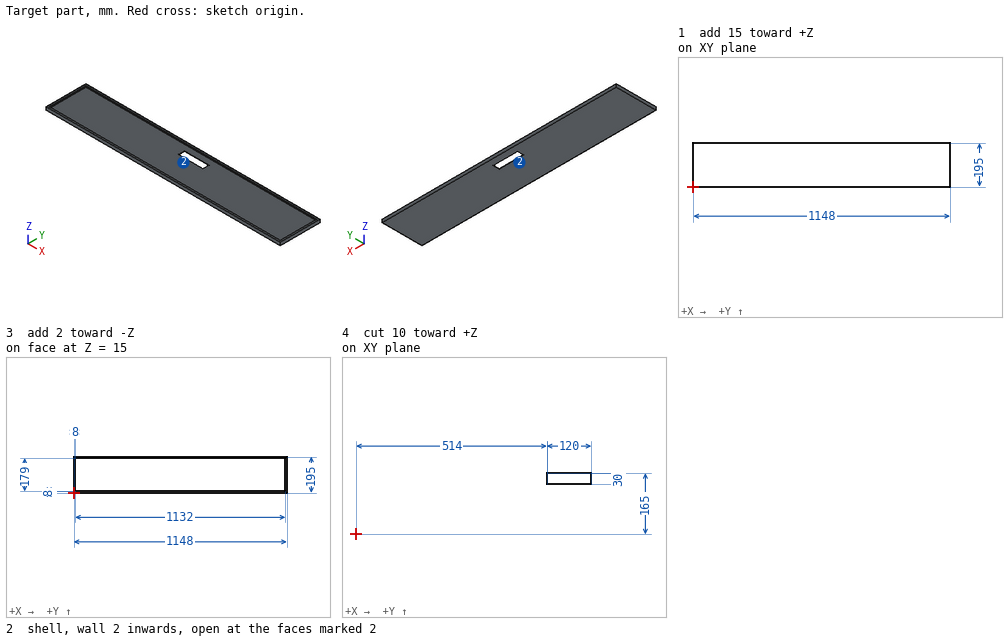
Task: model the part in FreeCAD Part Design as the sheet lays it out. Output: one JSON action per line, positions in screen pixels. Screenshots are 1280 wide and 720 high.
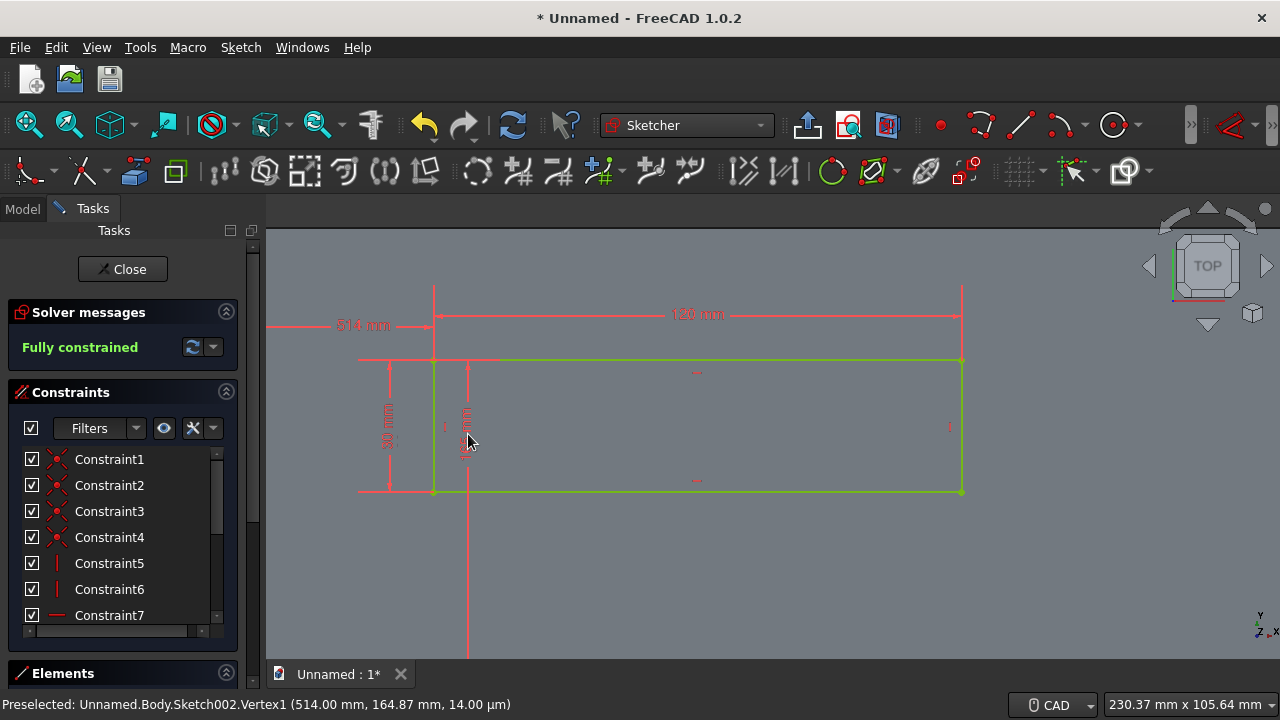
{"action": "left_click", "coordinate": [123, 269]}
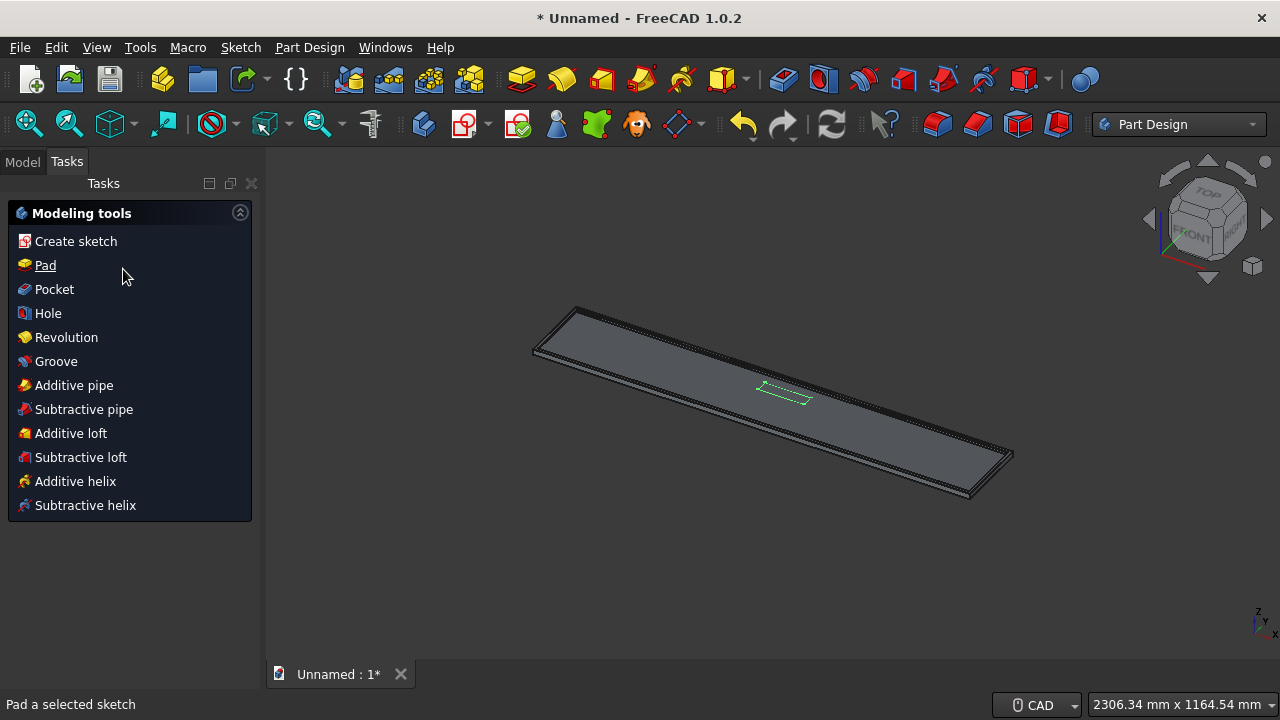
{"action": "left_click", "coordinate": [784, 80]}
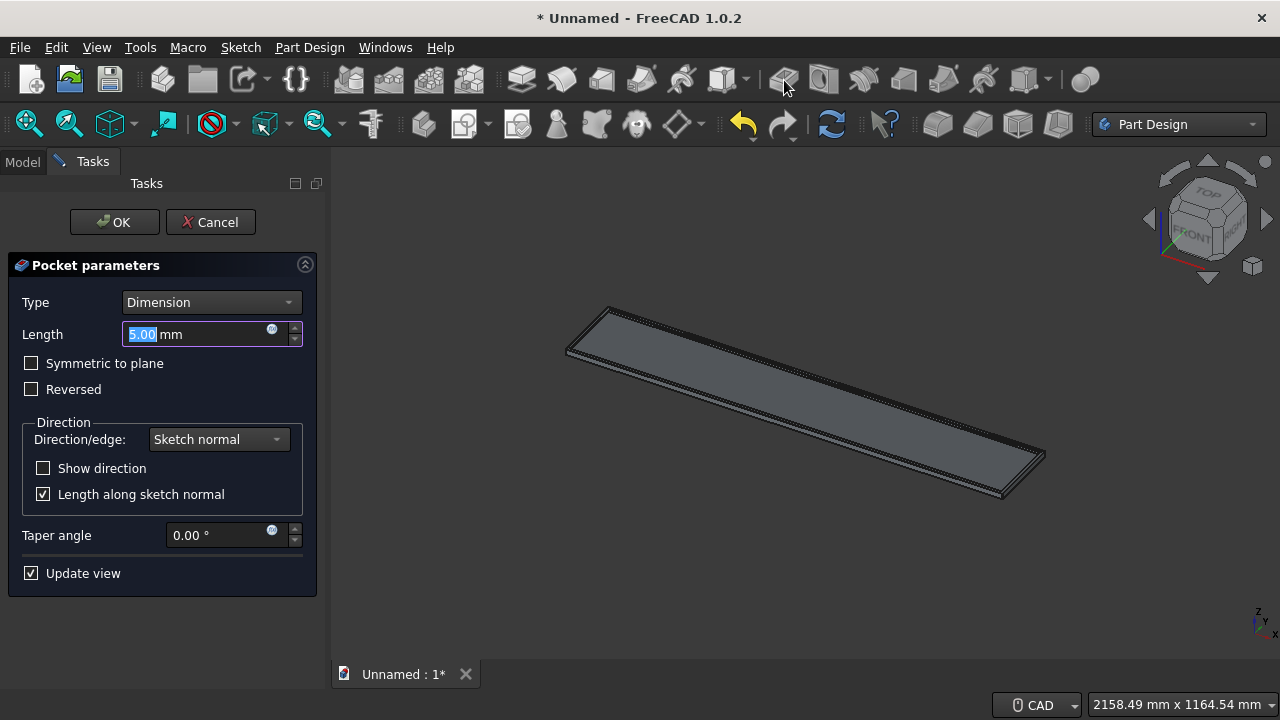
{"action": "type", "text": "10"}
{"action": "key", "text": "Tab"}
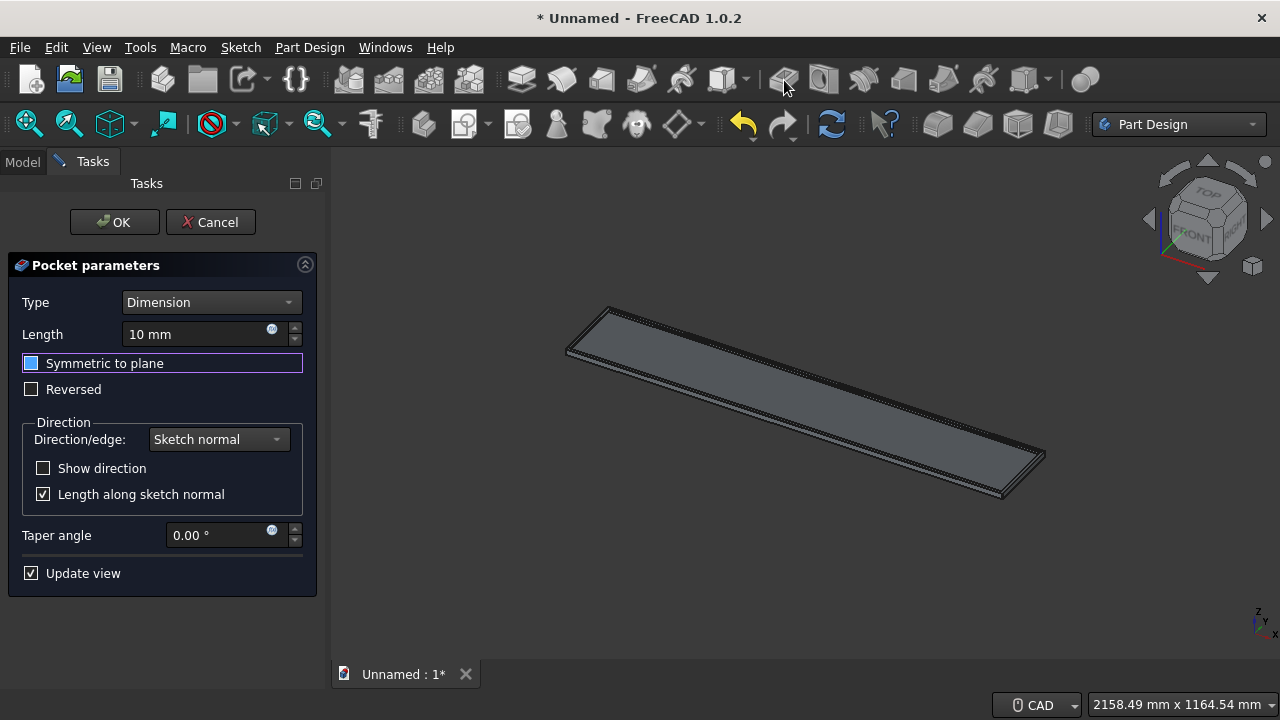
{"action": "left_click", "coordinate": [30, 389]}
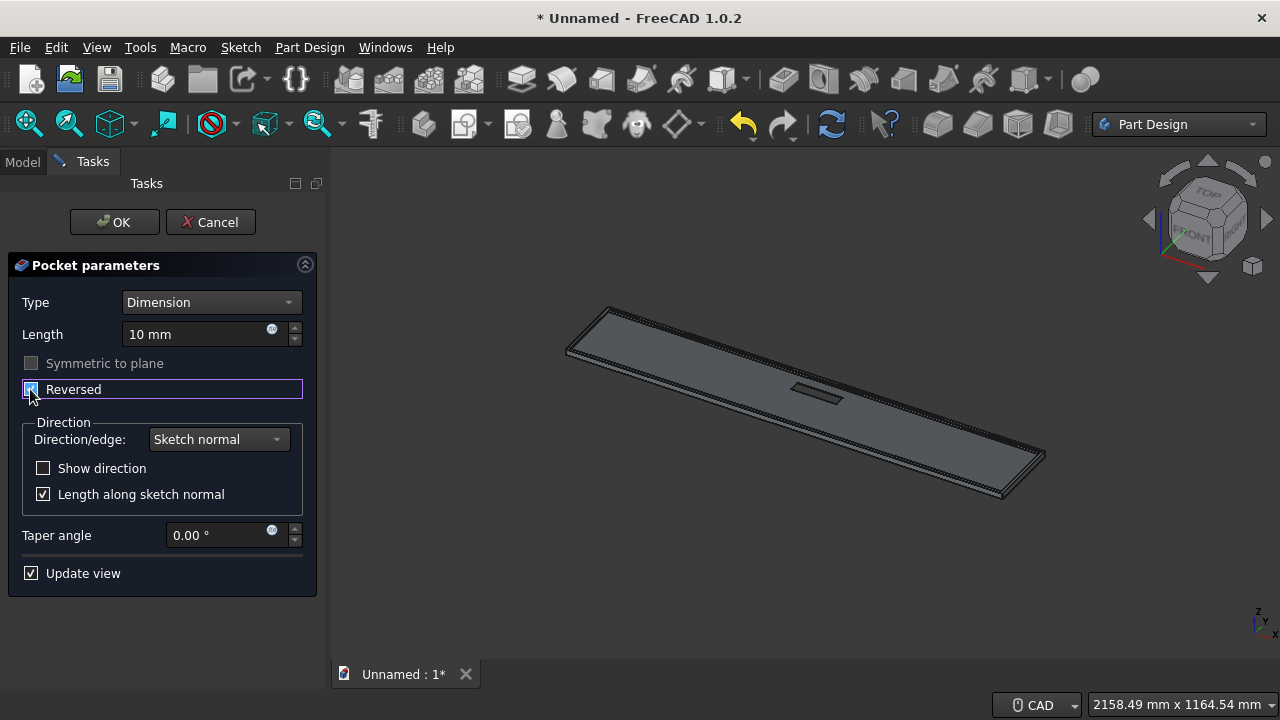
{"action": "left_click", "coordinate": [115, 222]}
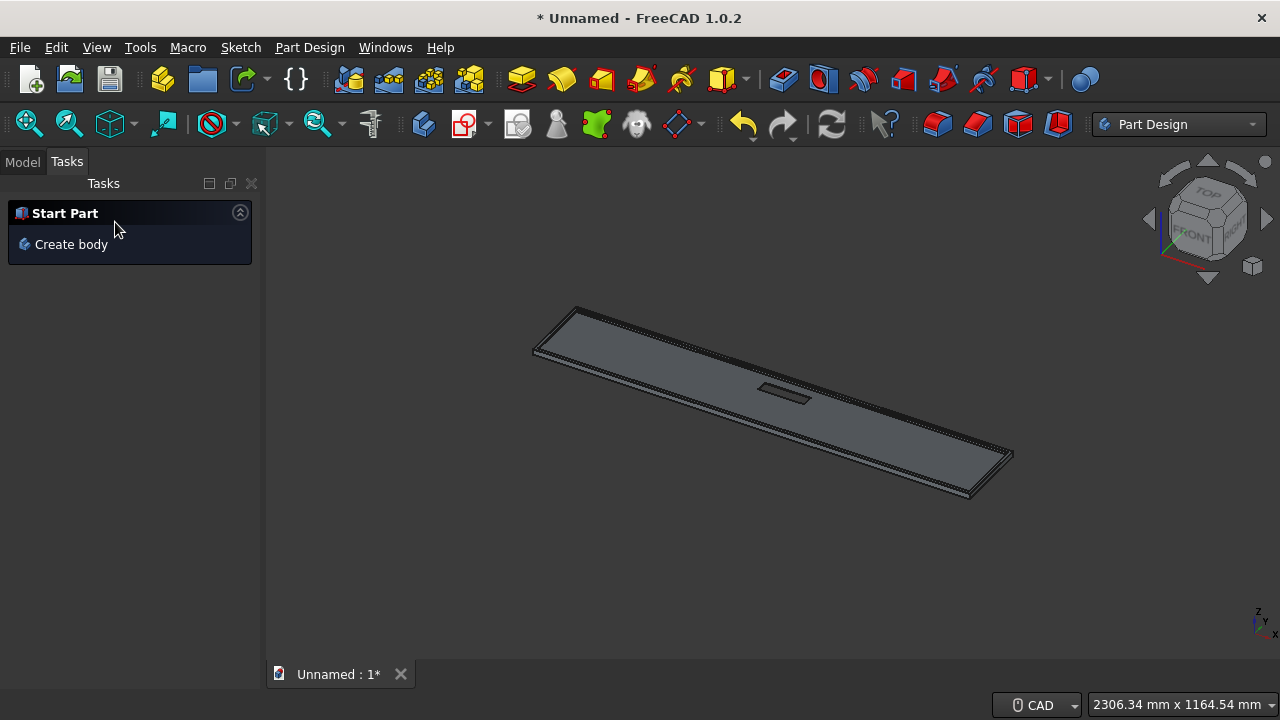
{"action": "key", "text": "0"}